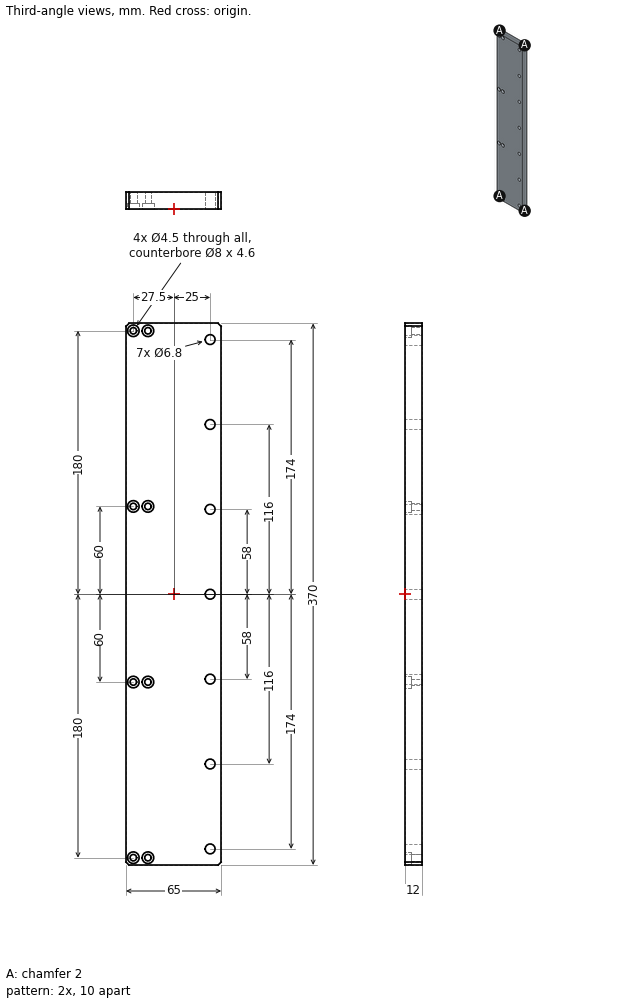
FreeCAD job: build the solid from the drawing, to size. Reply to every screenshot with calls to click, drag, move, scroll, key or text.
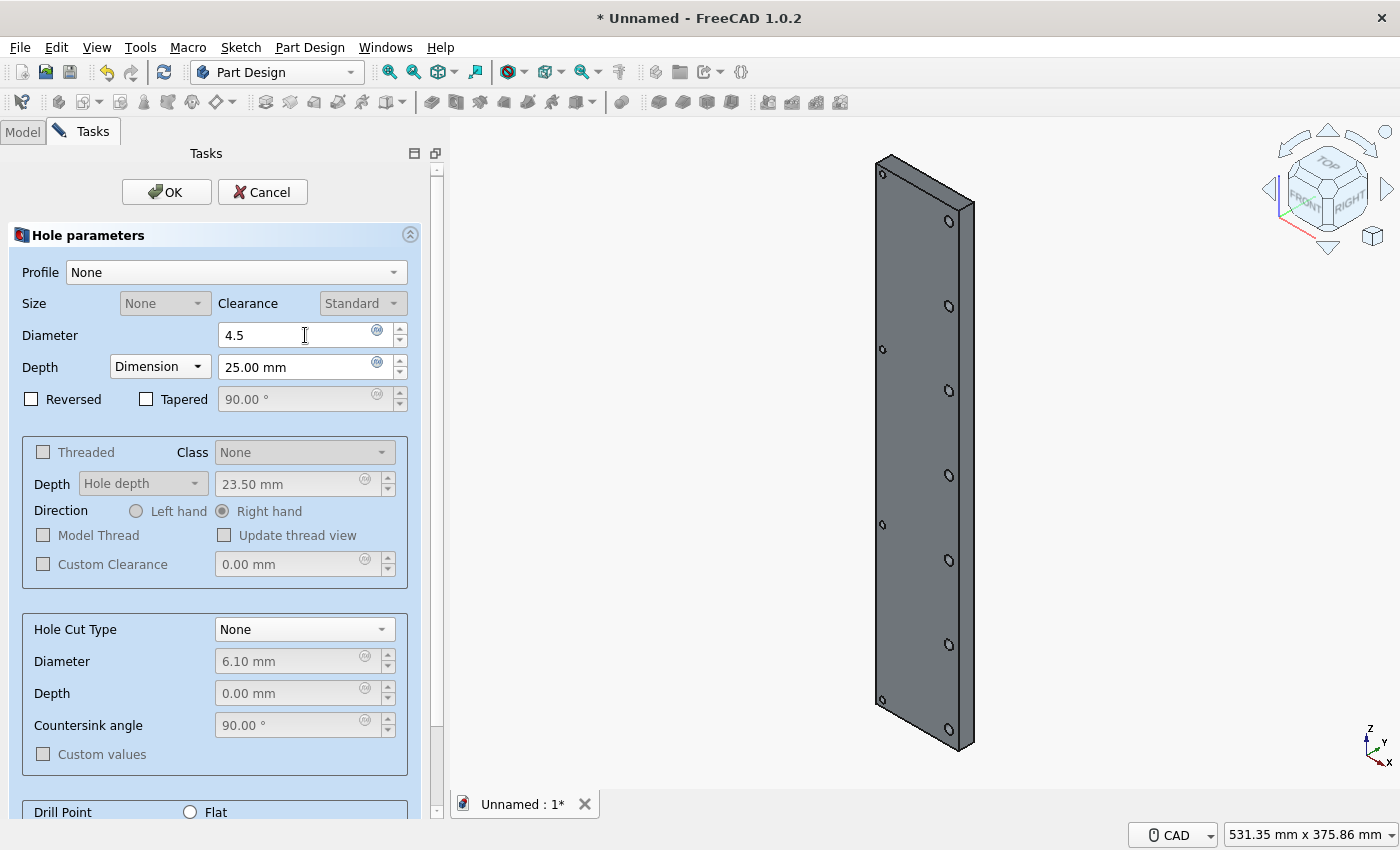
click(161, 366)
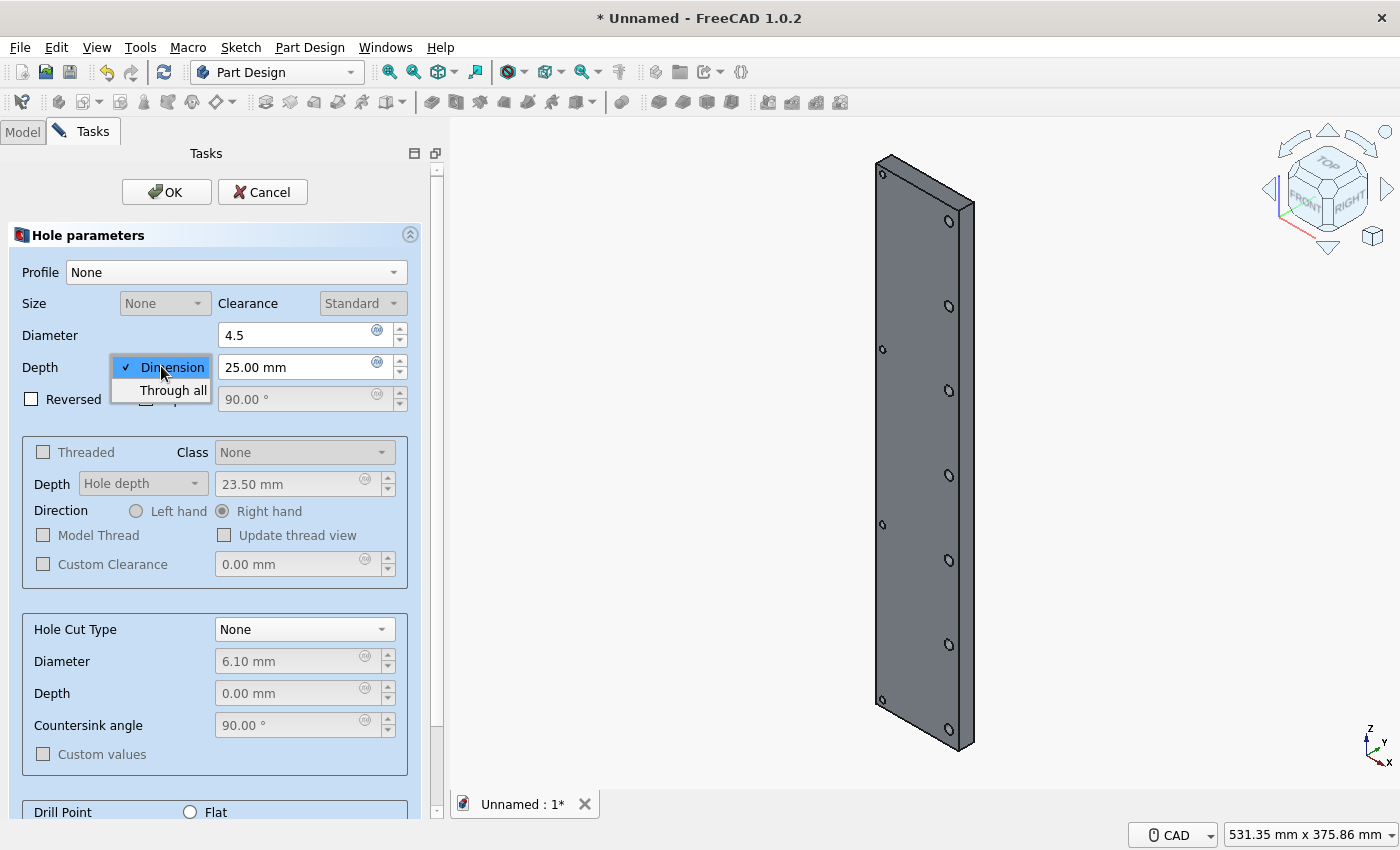
click(160, 390)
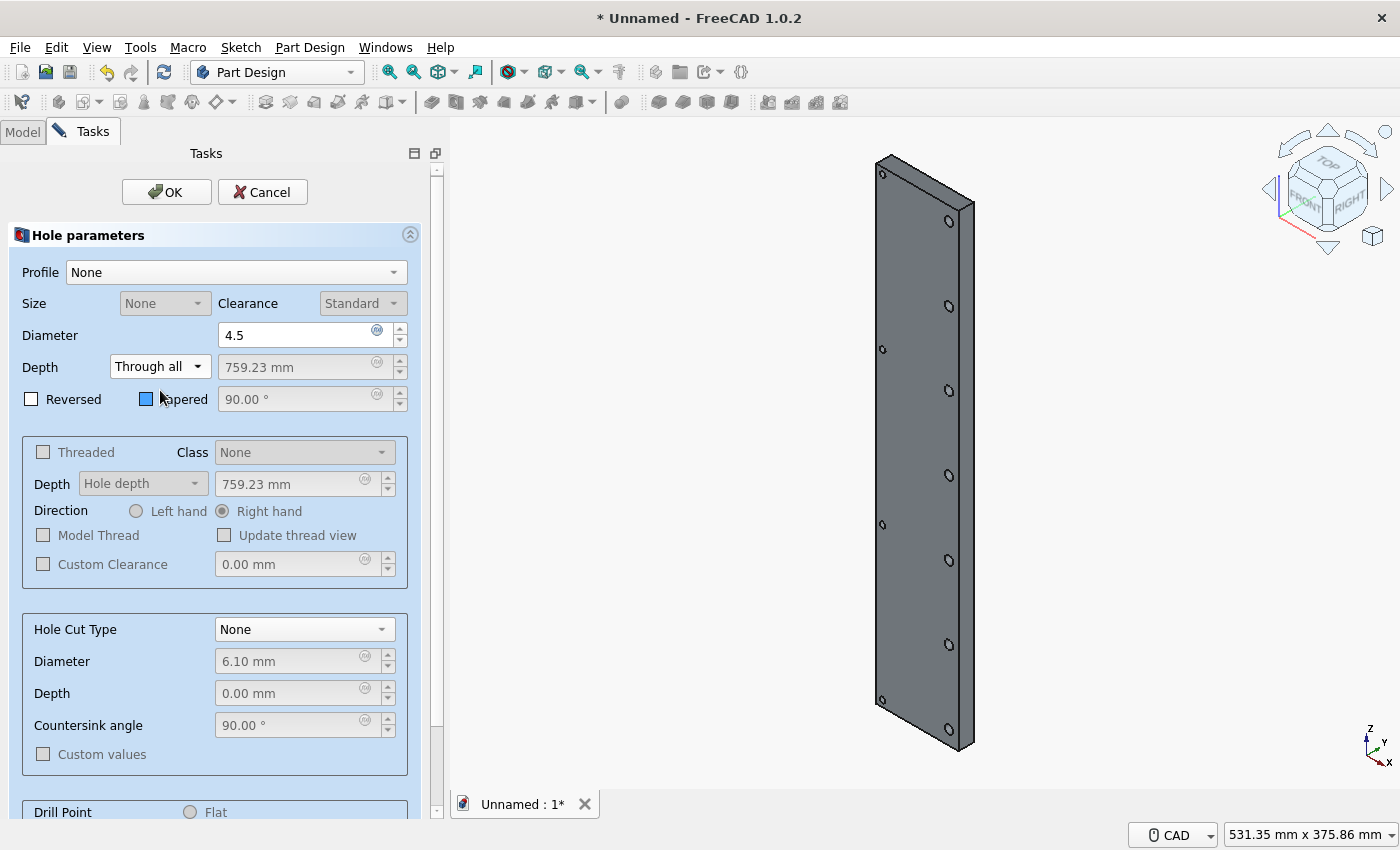
click(306, 630)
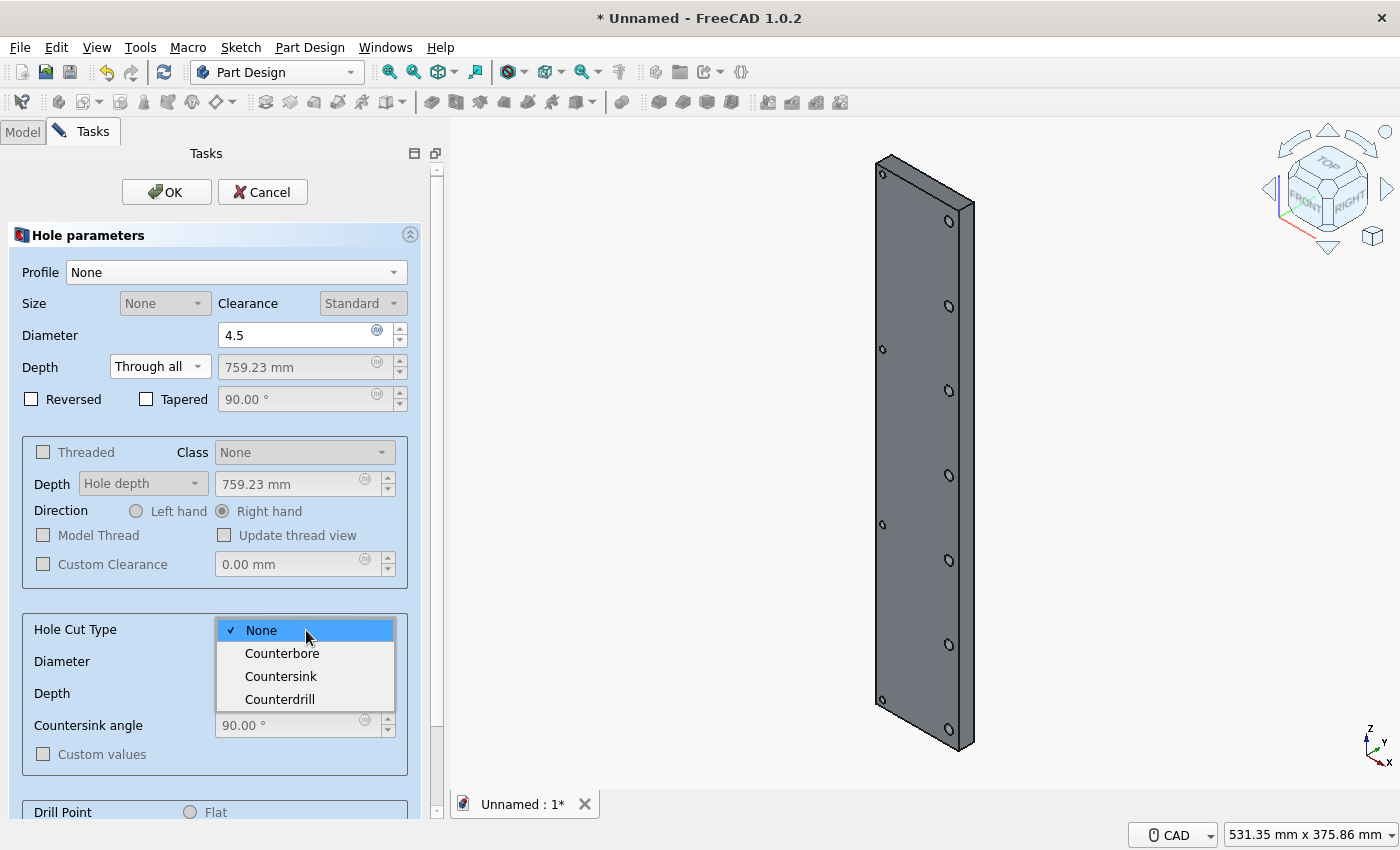
click(304, 654)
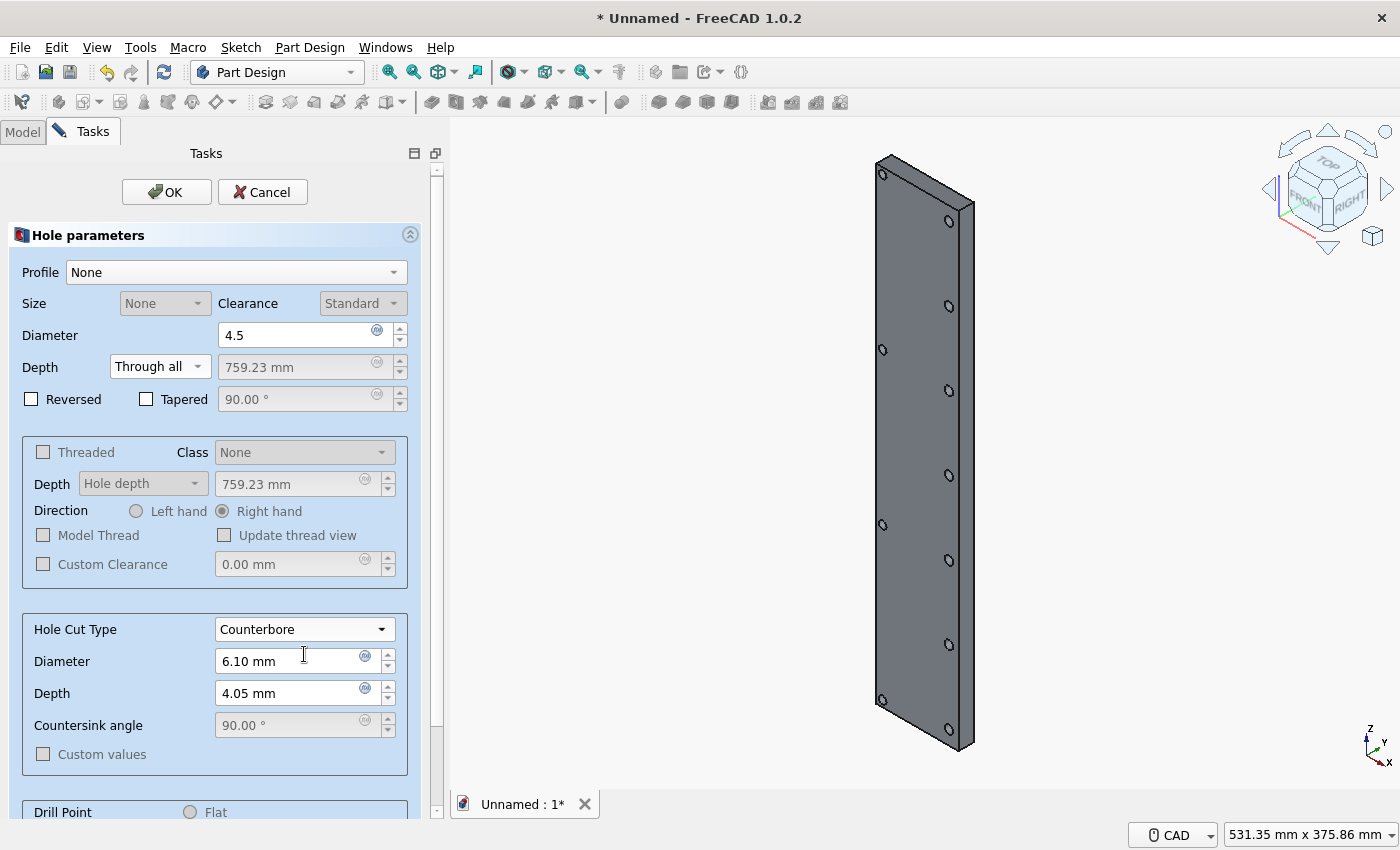
triple_click(298, 661)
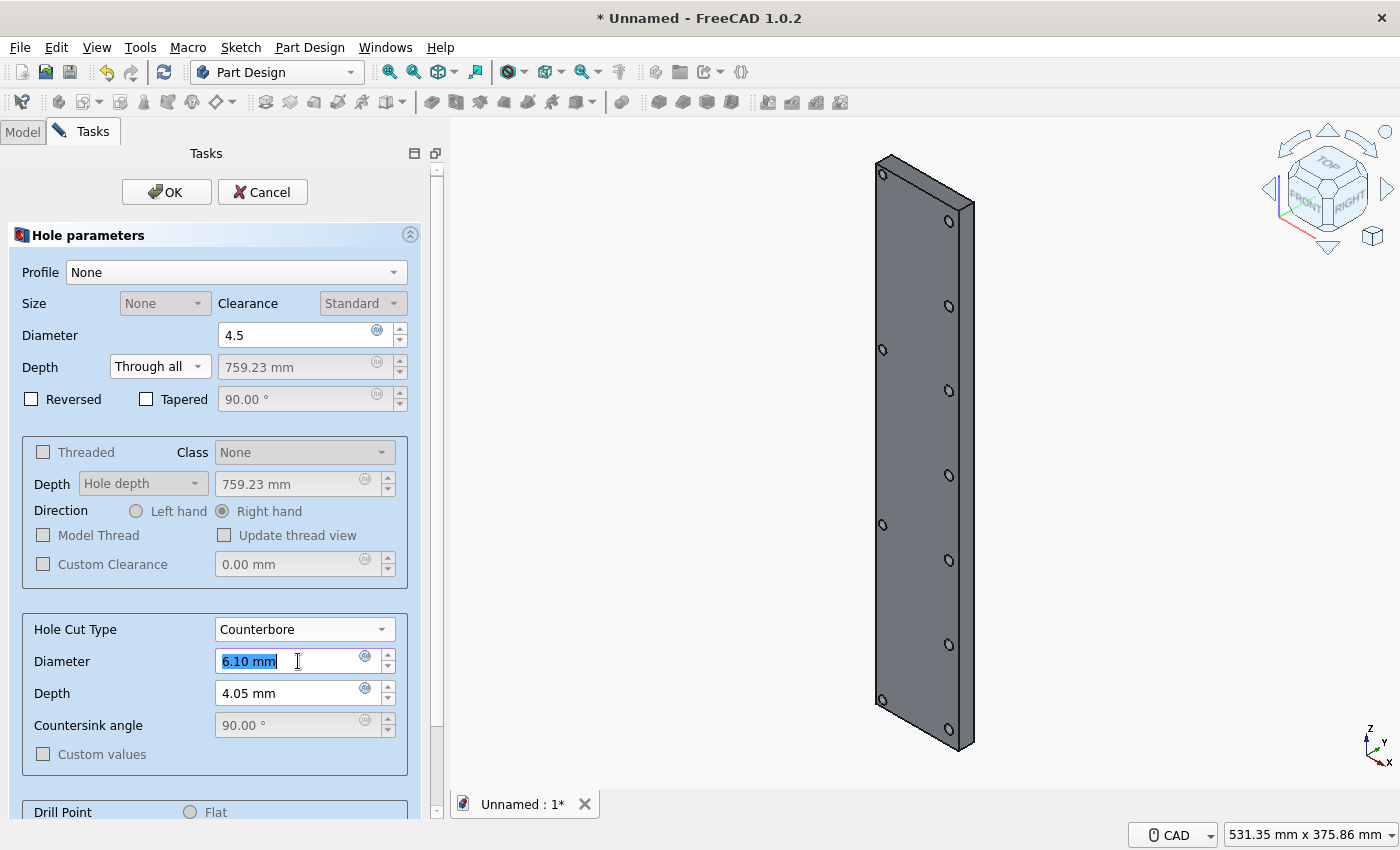
text(8)
key(Tab)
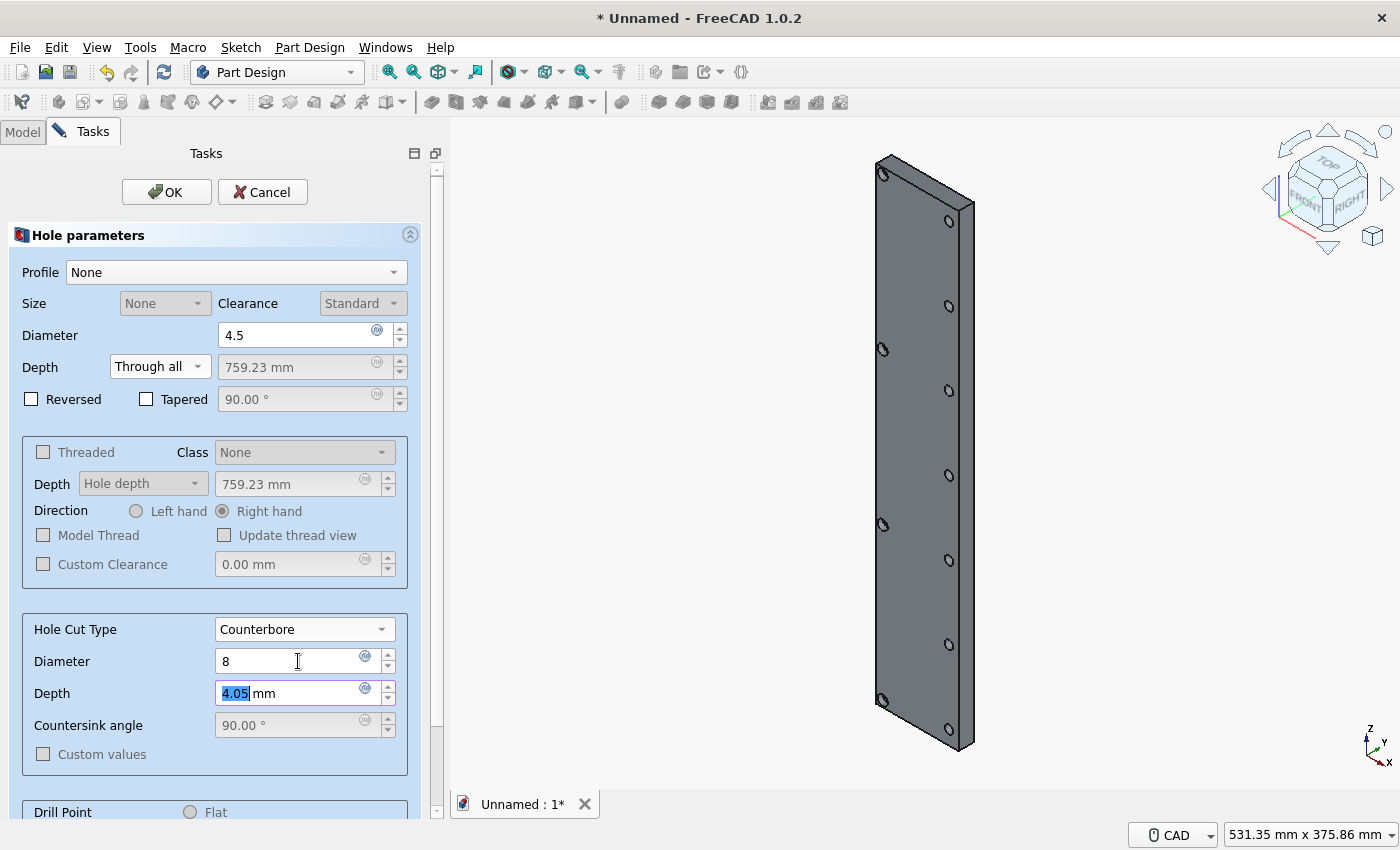
text(4.6)
key(Tab)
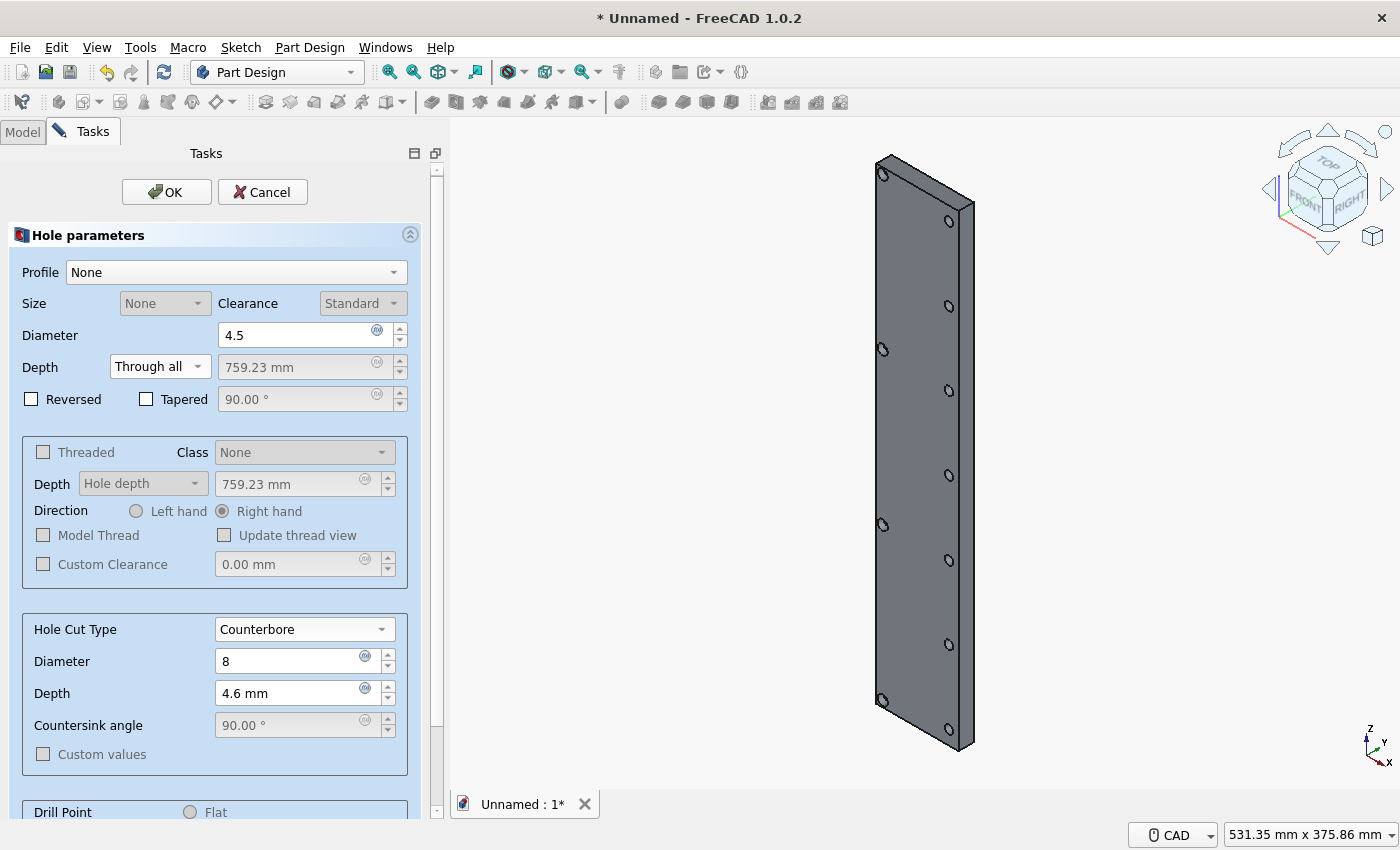
click(167, 192)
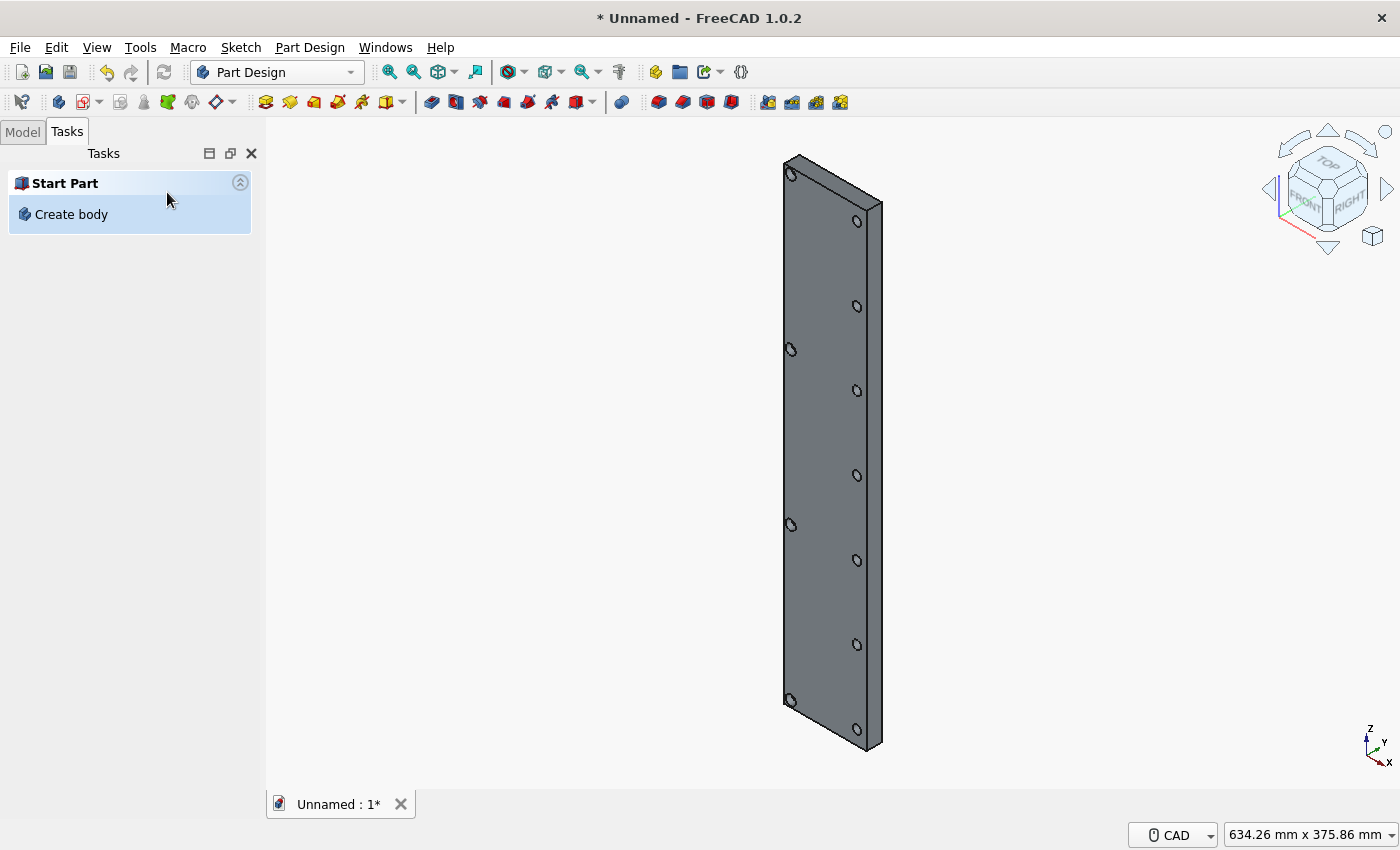
click(874, 206)